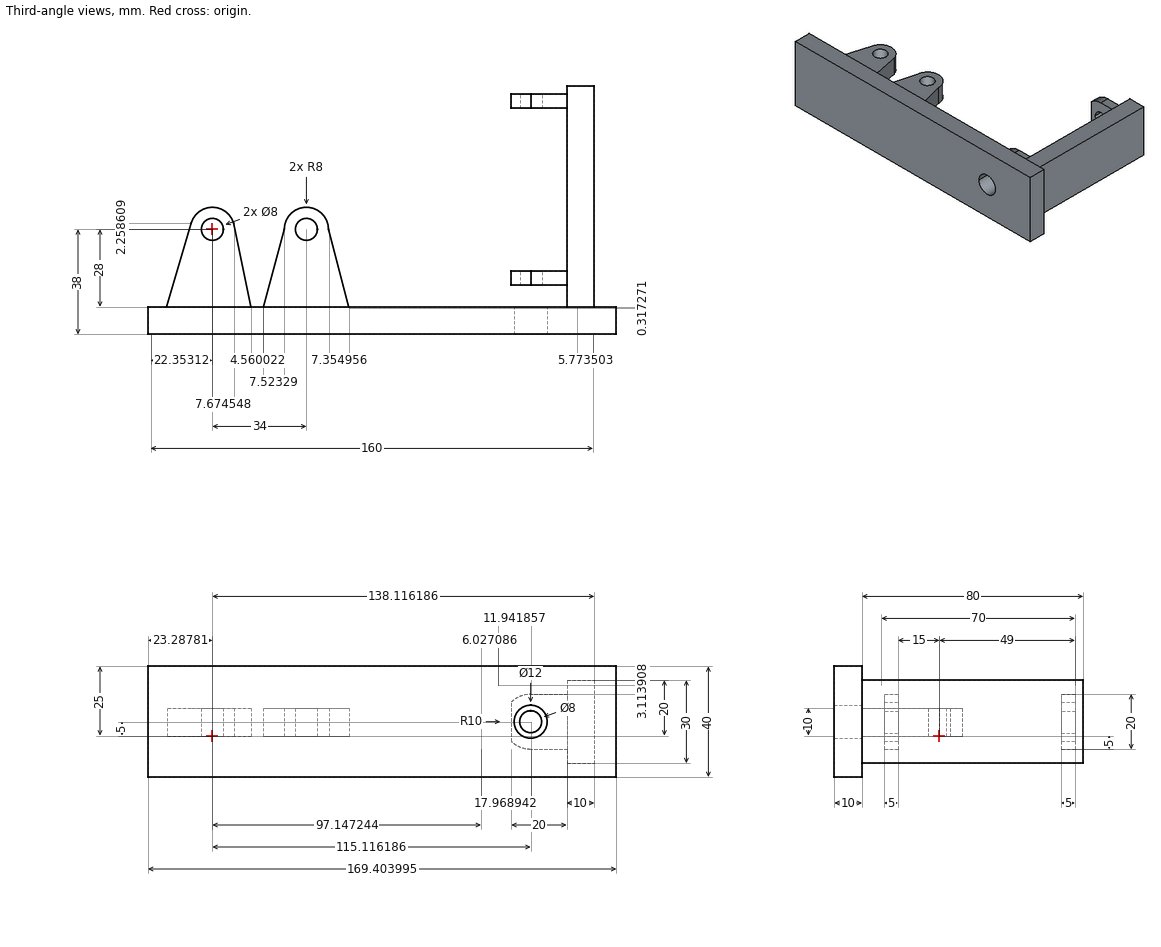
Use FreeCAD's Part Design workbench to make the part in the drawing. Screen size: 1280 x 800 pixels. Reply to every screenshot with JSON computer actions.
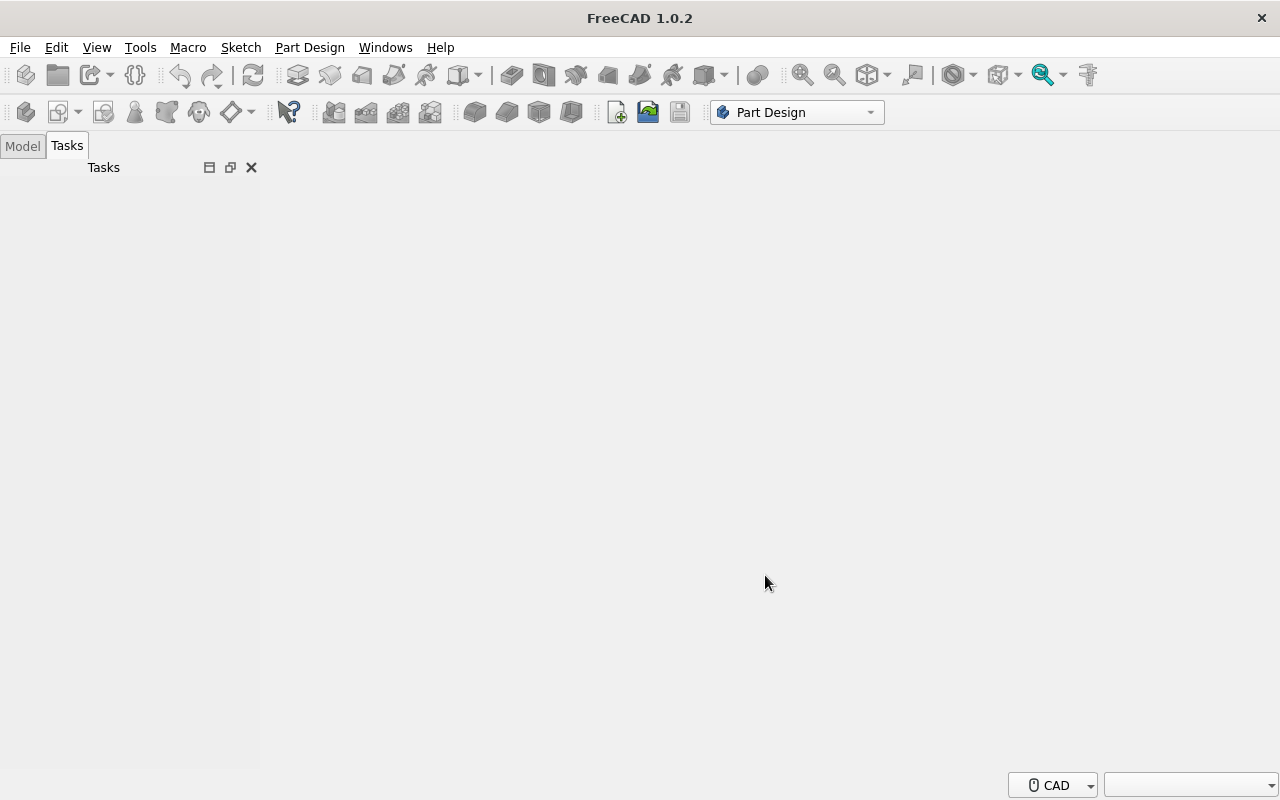
{"action": "left_click", "coordinate": [616, 112]}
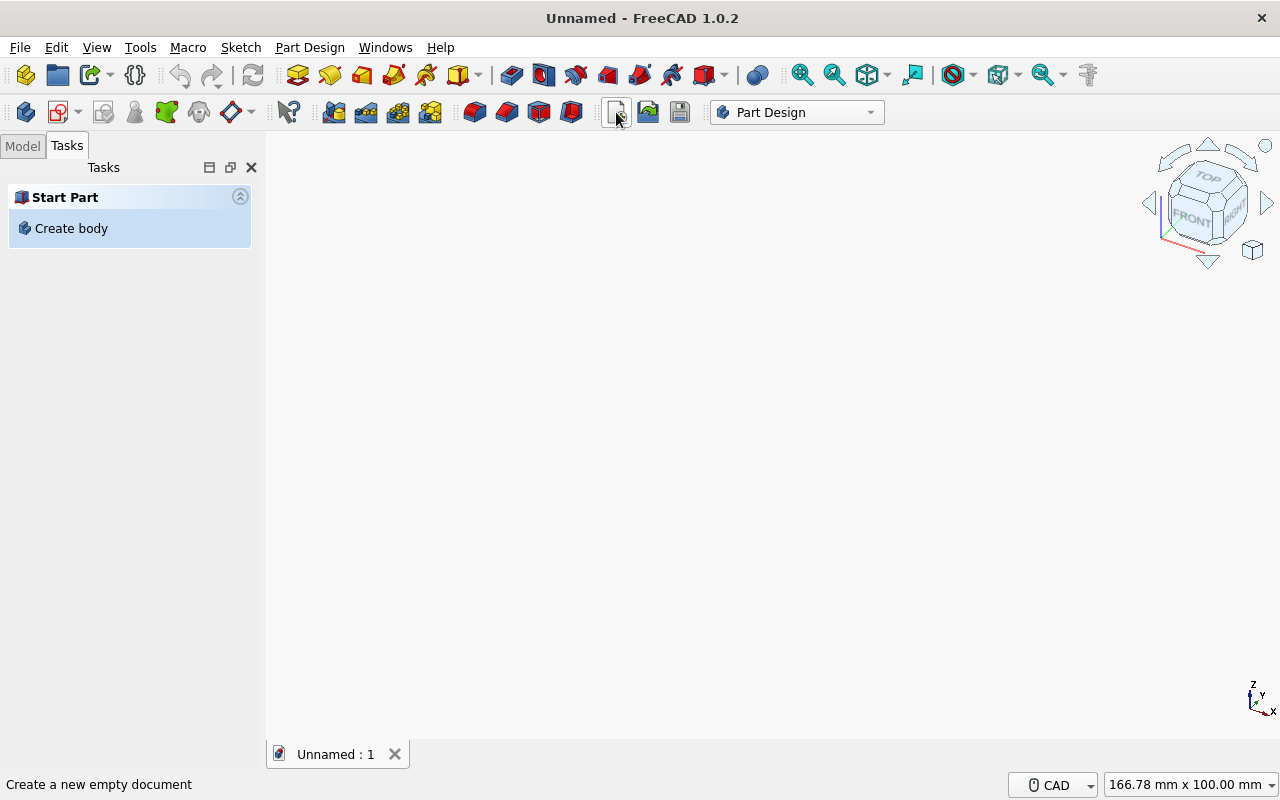
{"action": "left_click", "coordinate": [58, 112]}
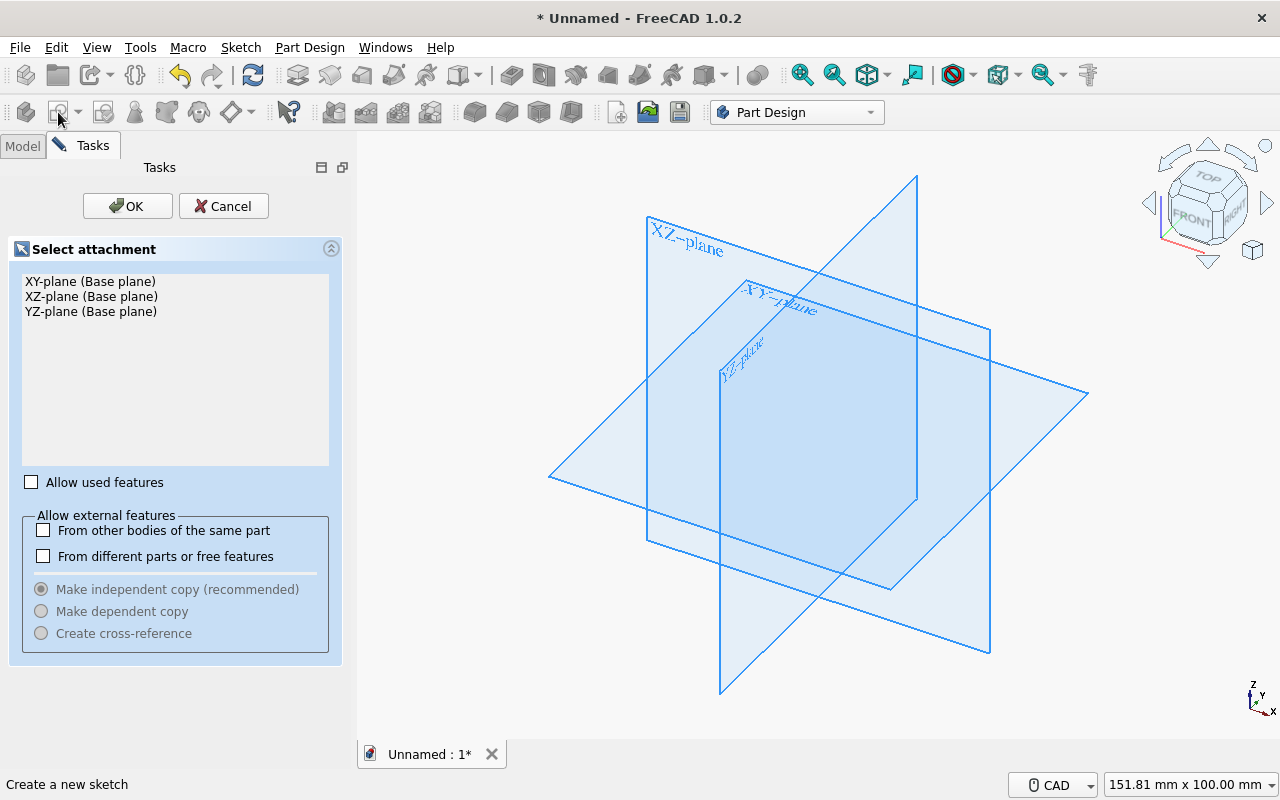
{"action": "left_click", "coordinate": [82, 282]}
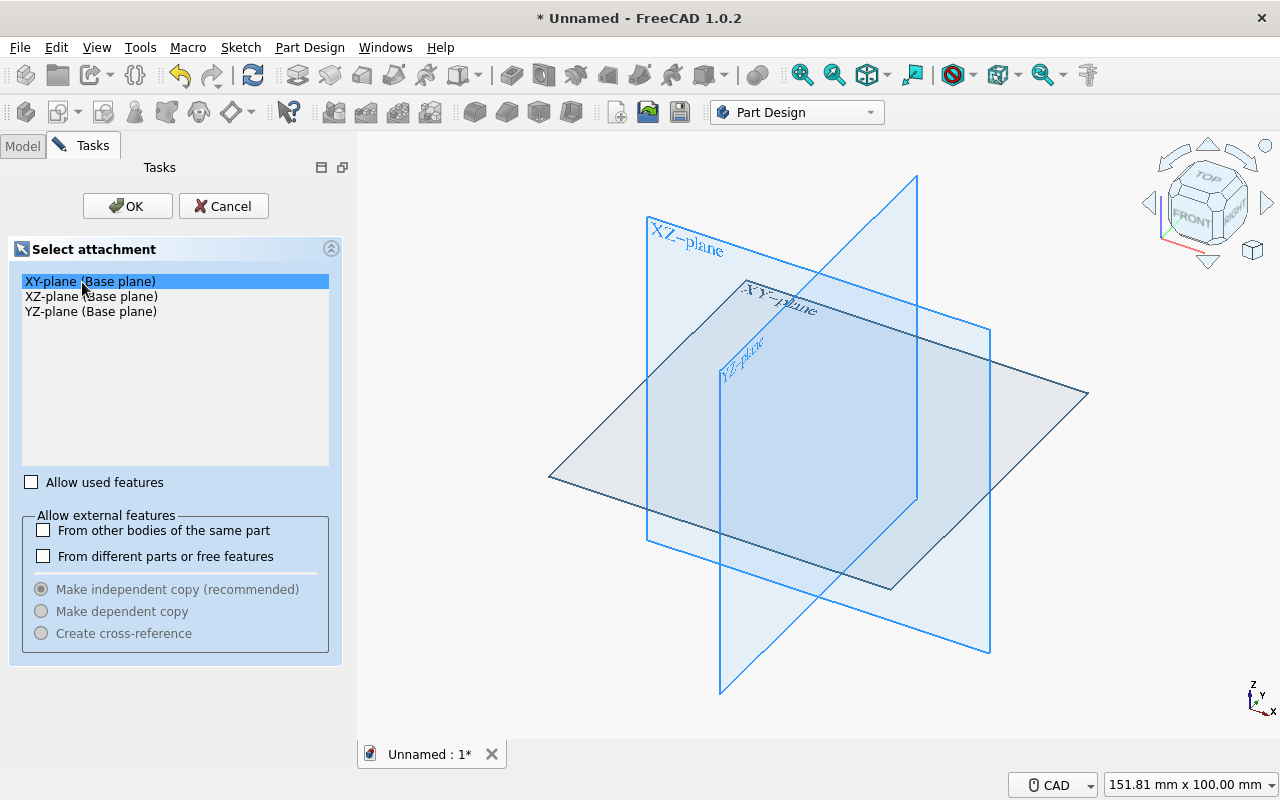
{"action": "left_click", "coordinate": [128, 206]}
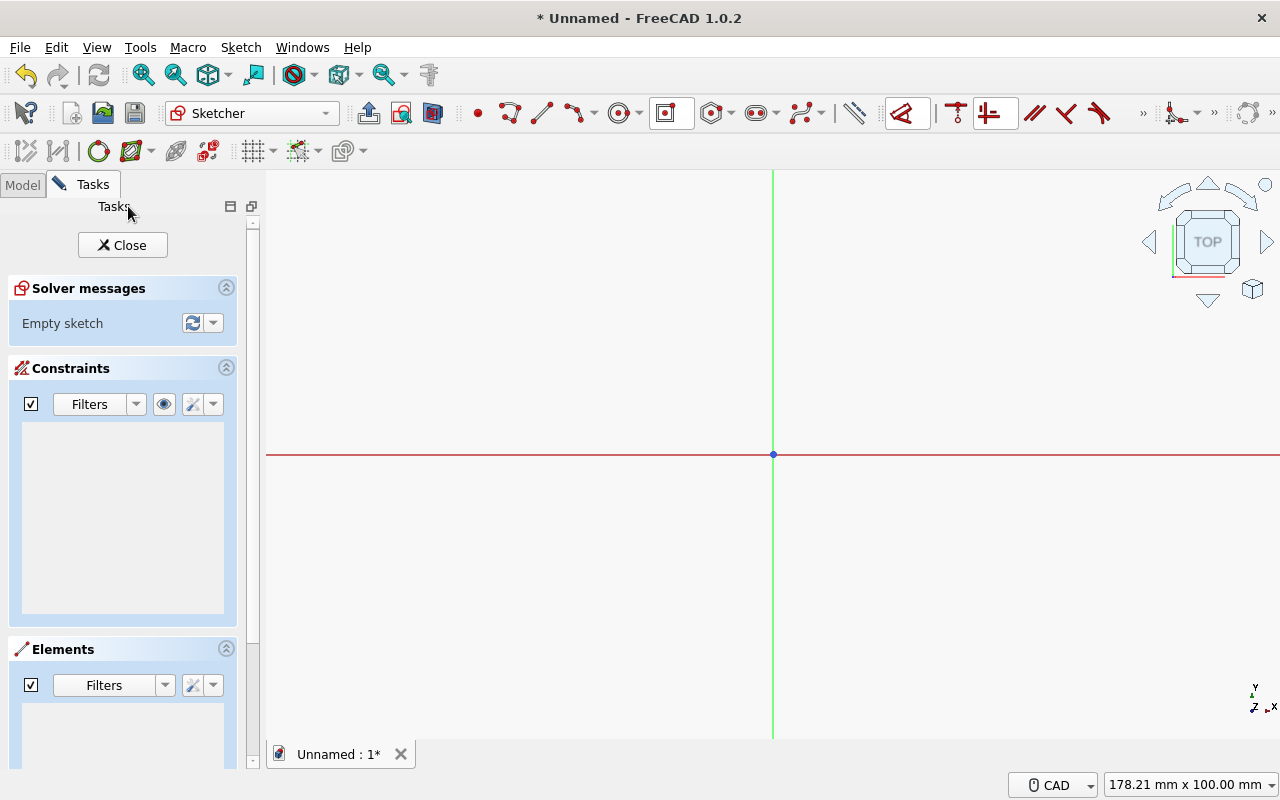
{"action": "scroll", "coordinate": [294, 351], "scroll_direction": "down", "scroll_amount": 3}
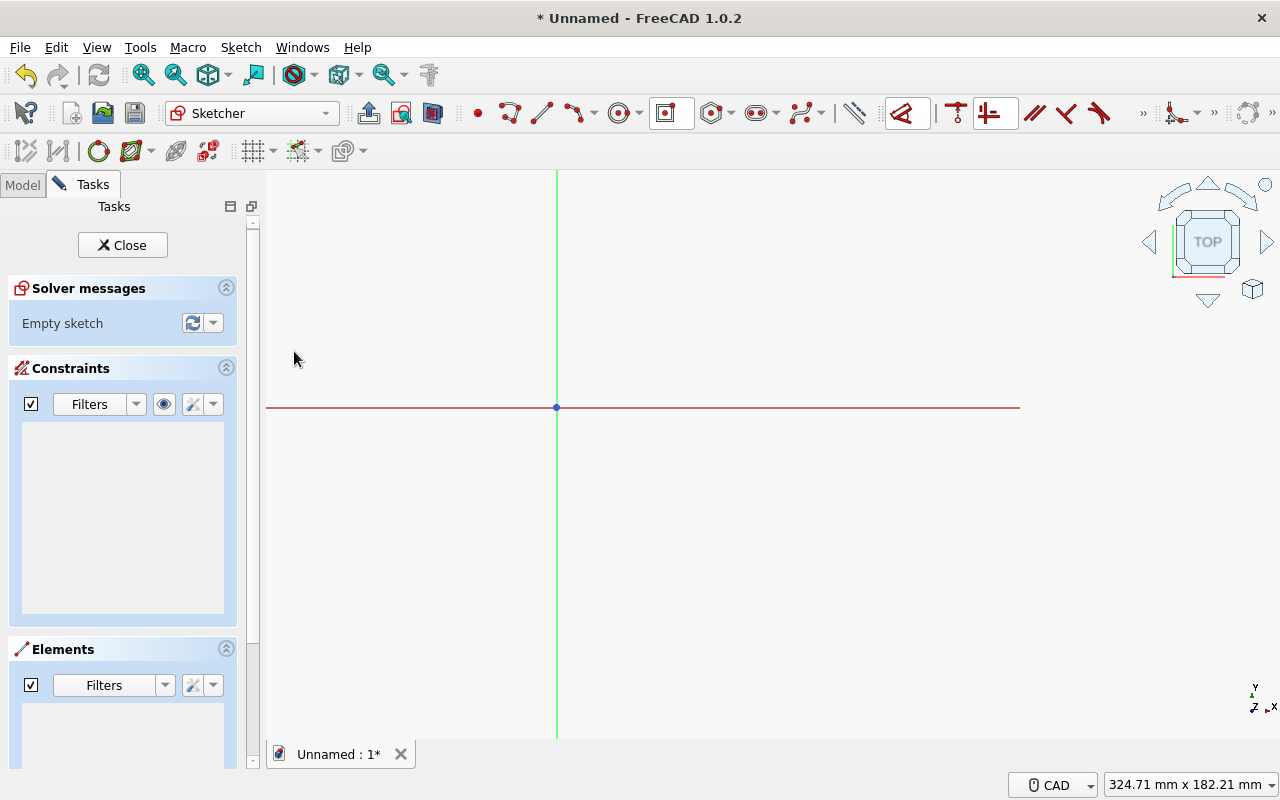
{"action": "left_click", "coordinate": [510, 114]}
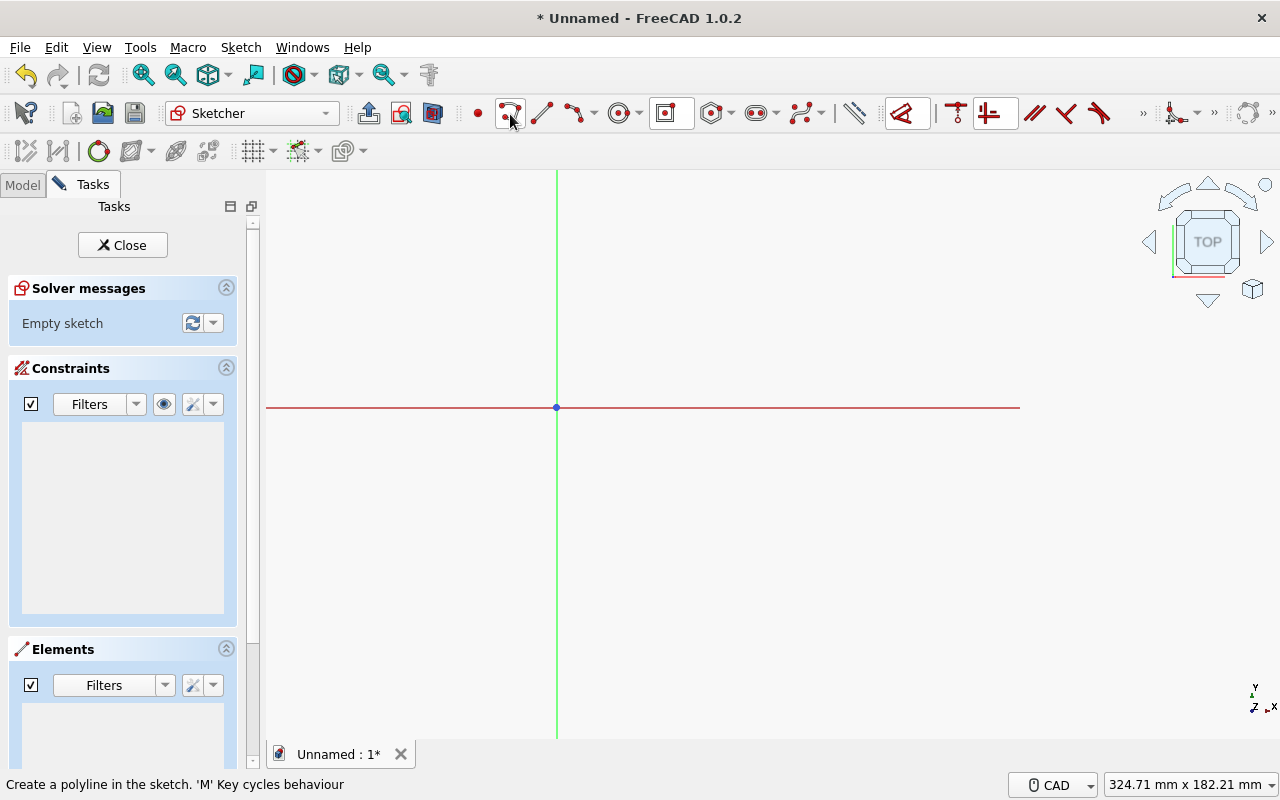
{"action": "scroll", "coordinate": [533, 401], "scroll_direction": "up", "scroll_amount": 5}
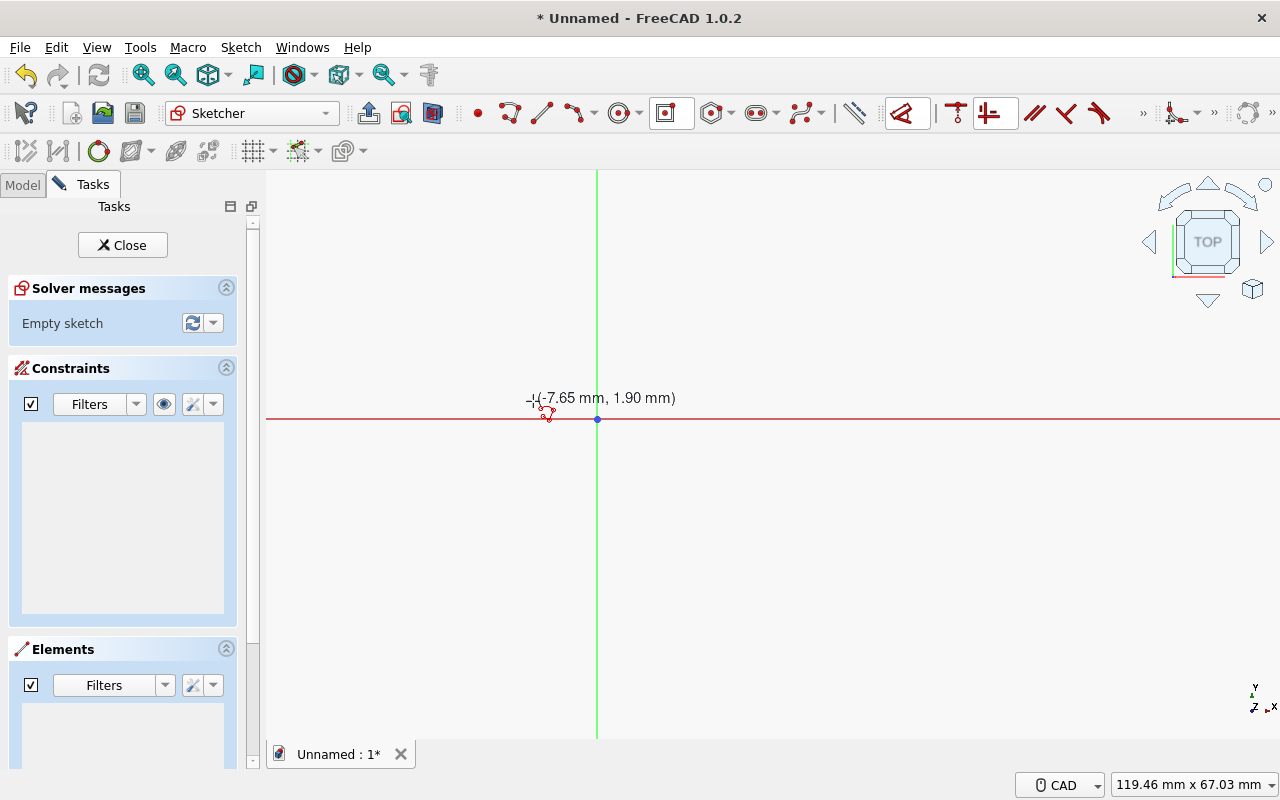
{"action": "left_click", "coordinate": [532, 400]}
{"action": "left_click", "coordinate": [457, 657]}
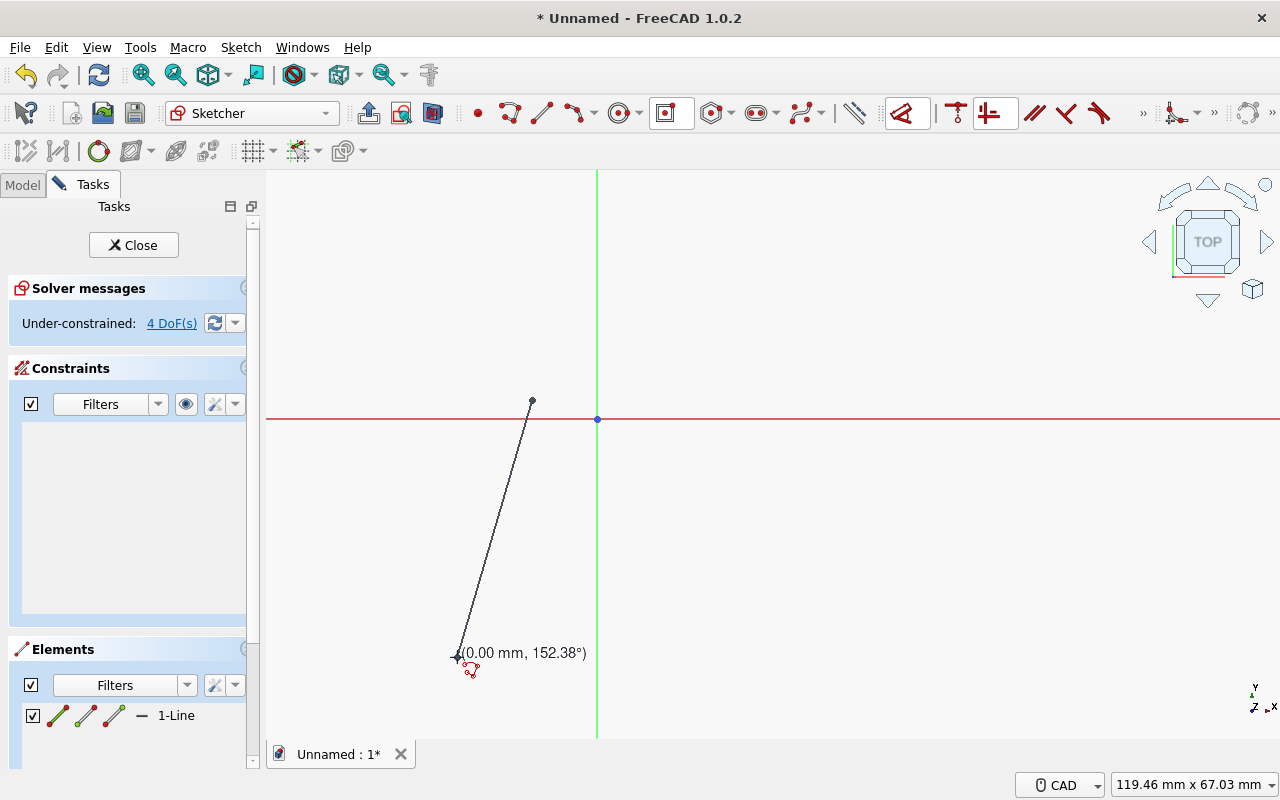
{"action": "scroll", "coordinate": [393, 379], "scroll_direction": "down", "scroll_amount": 4}